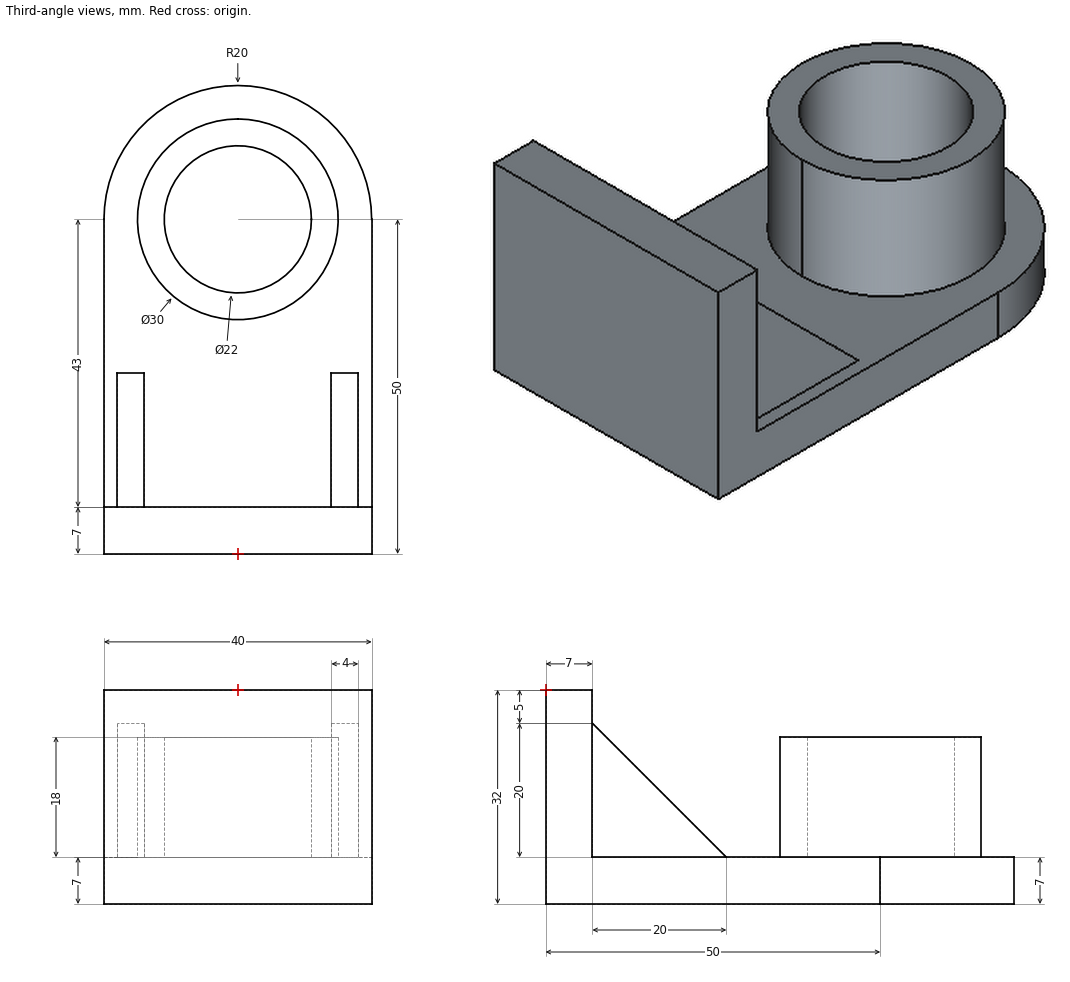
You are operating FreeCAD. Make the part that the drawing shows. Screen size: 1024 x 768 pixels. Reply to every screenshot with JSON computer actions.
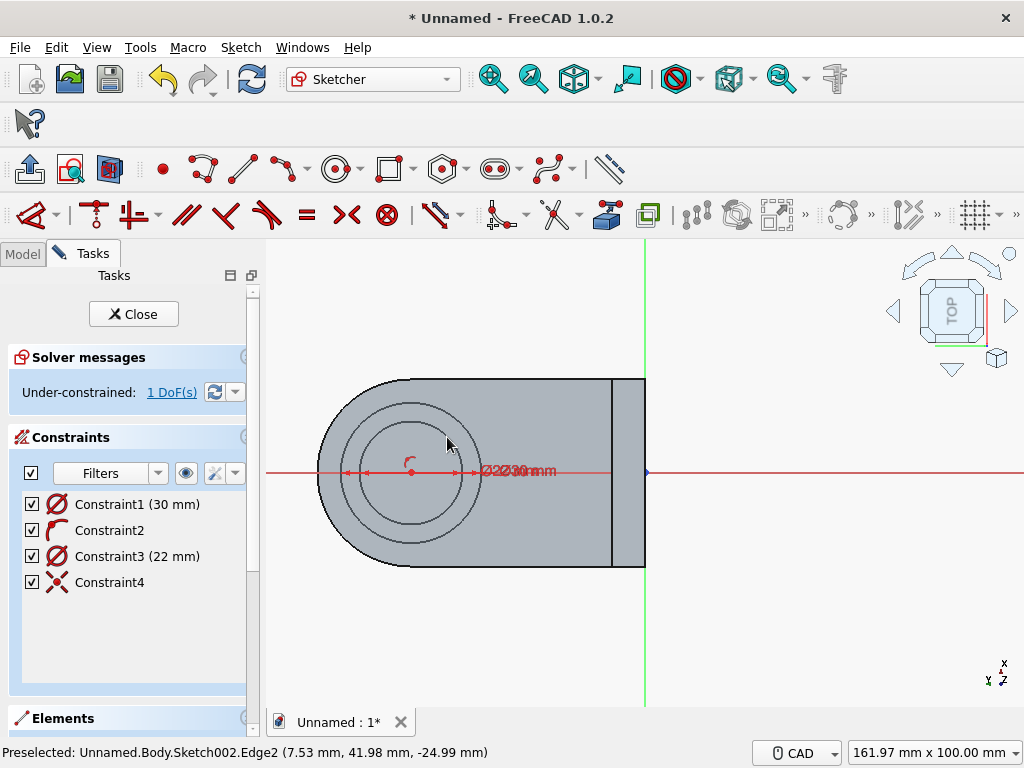
{"action": "left_click", "coordinate": [32, 216]}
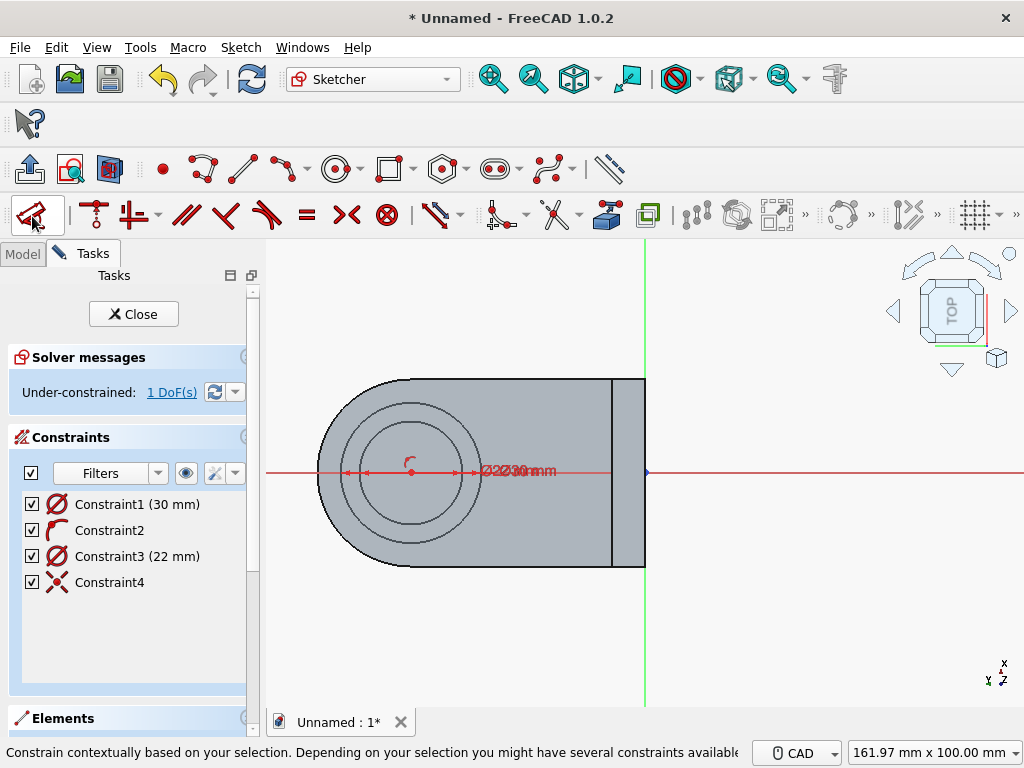
{"action": "left_click", "coordinate": [411, 473]}
{"action": "left_click", "coordinate": [528, 439]}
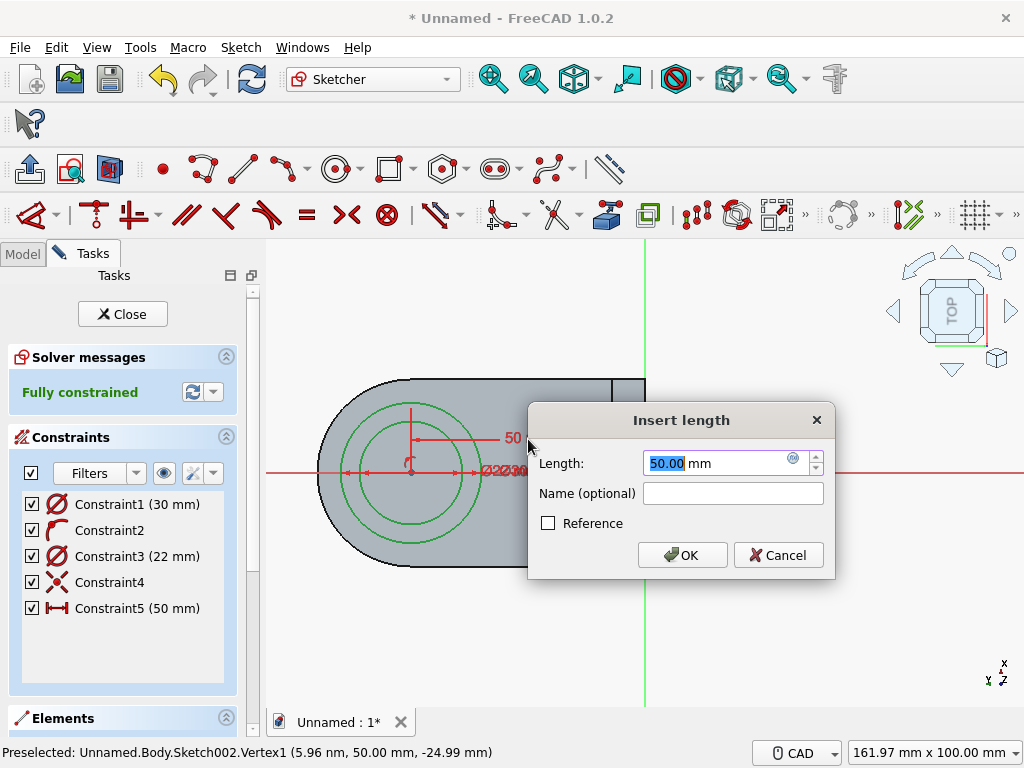
{"action": "type", "text": "50"}
{"action": "key", "text": "Return"}
{"action": "key", "text": "Escape"}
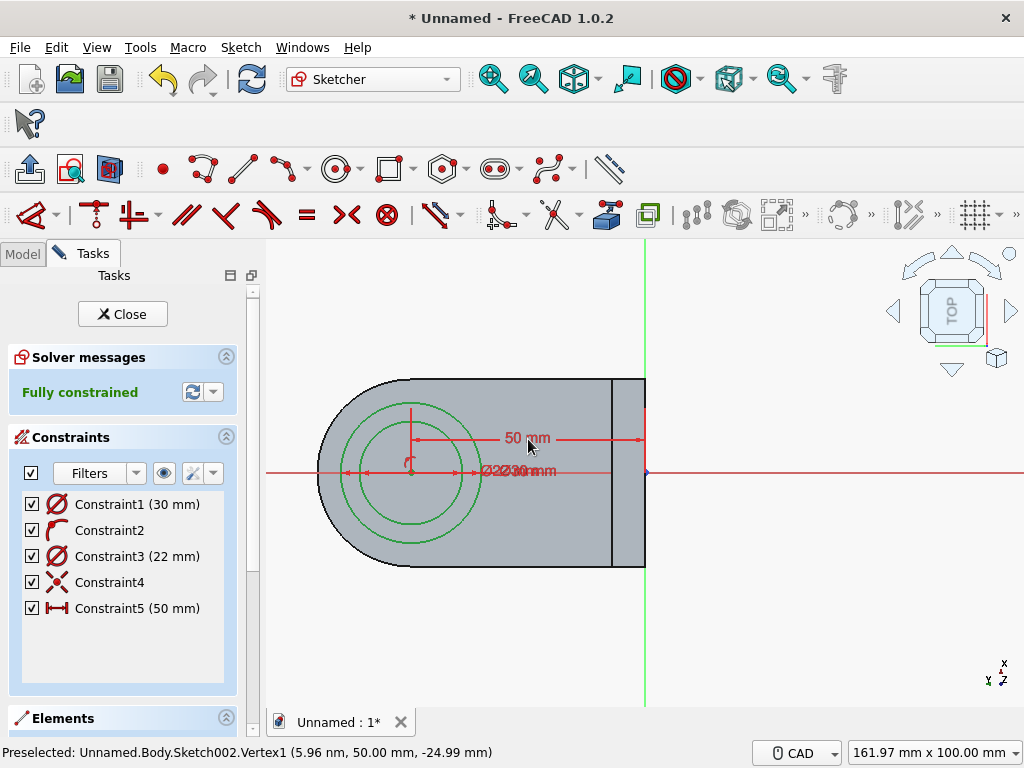
{"action": "left_click", "coordinate": [123, 314]}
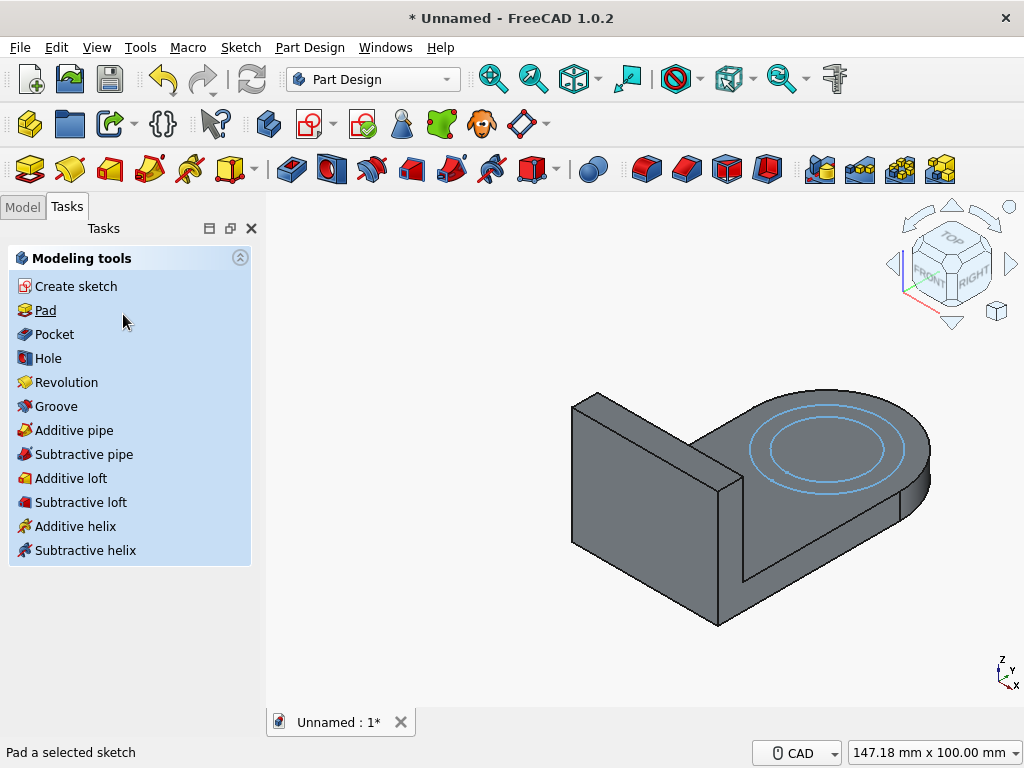
{"action": "left_click", "coordinate": [30, 170]}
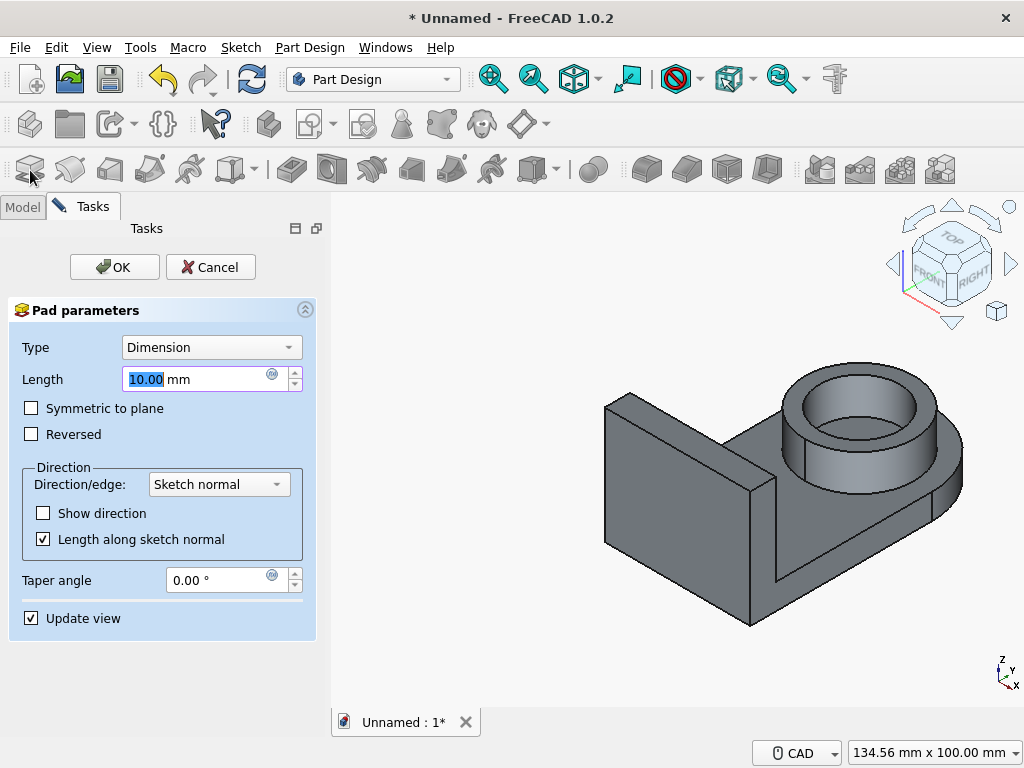
{"action": "type", "text": "18"}
{"action": "key", "text": "Tab"}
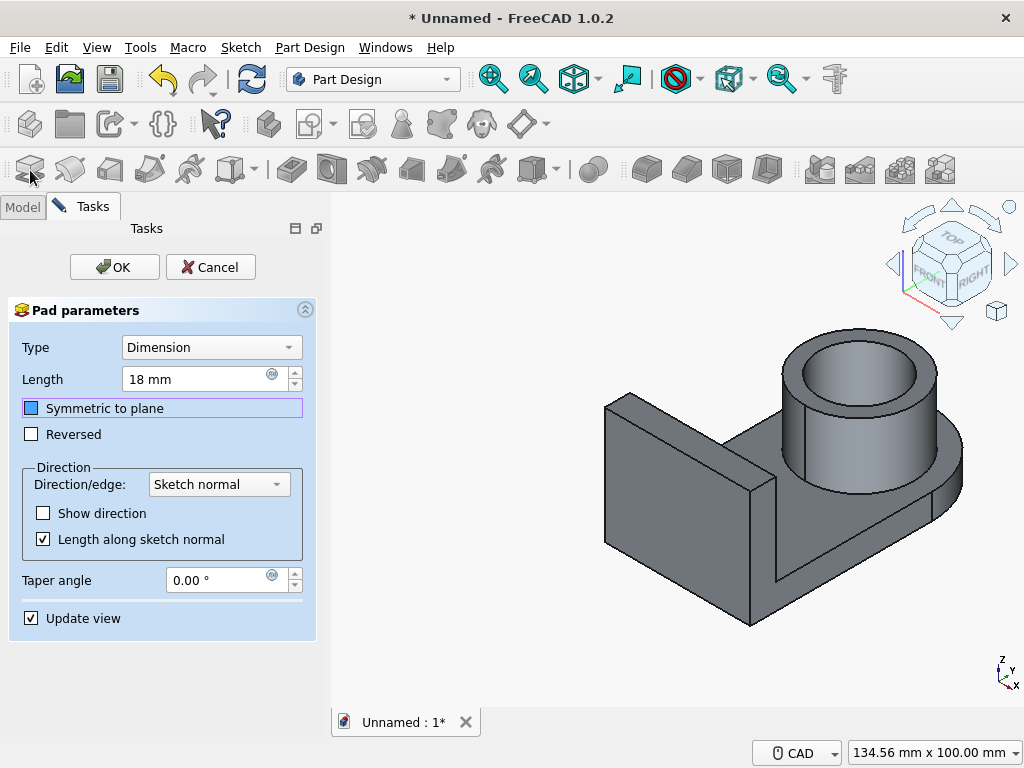
{"action": "left_click", "coordinate": [115, 267]}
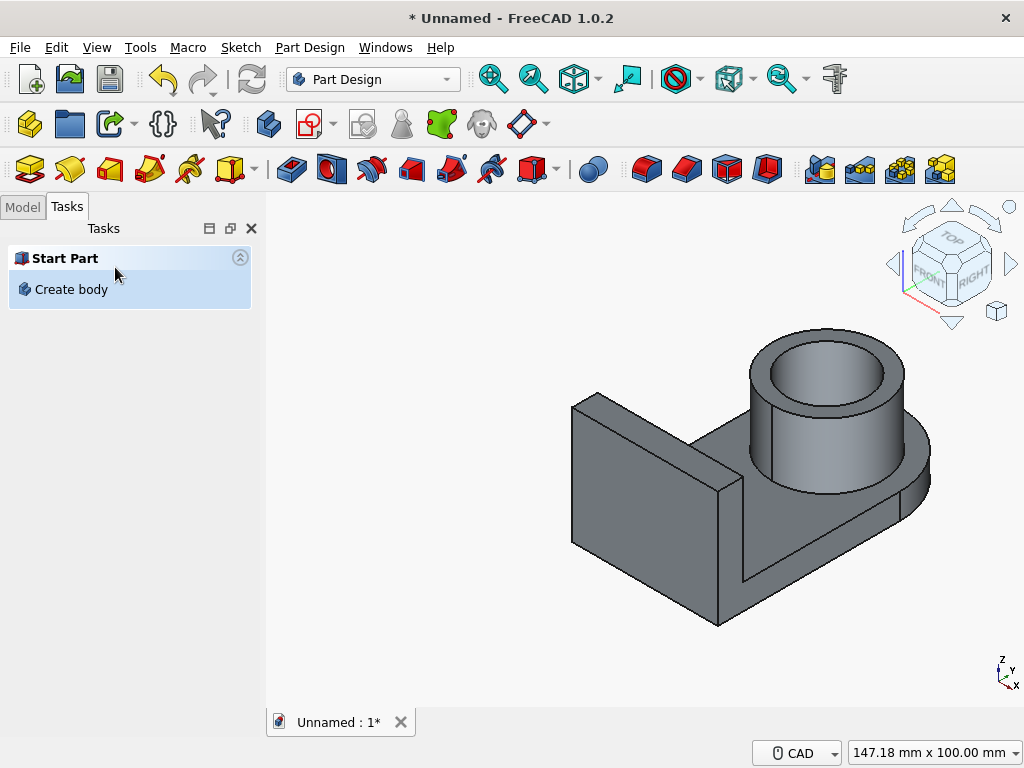
{"action": "left_click", "coordinate": [23, 206]}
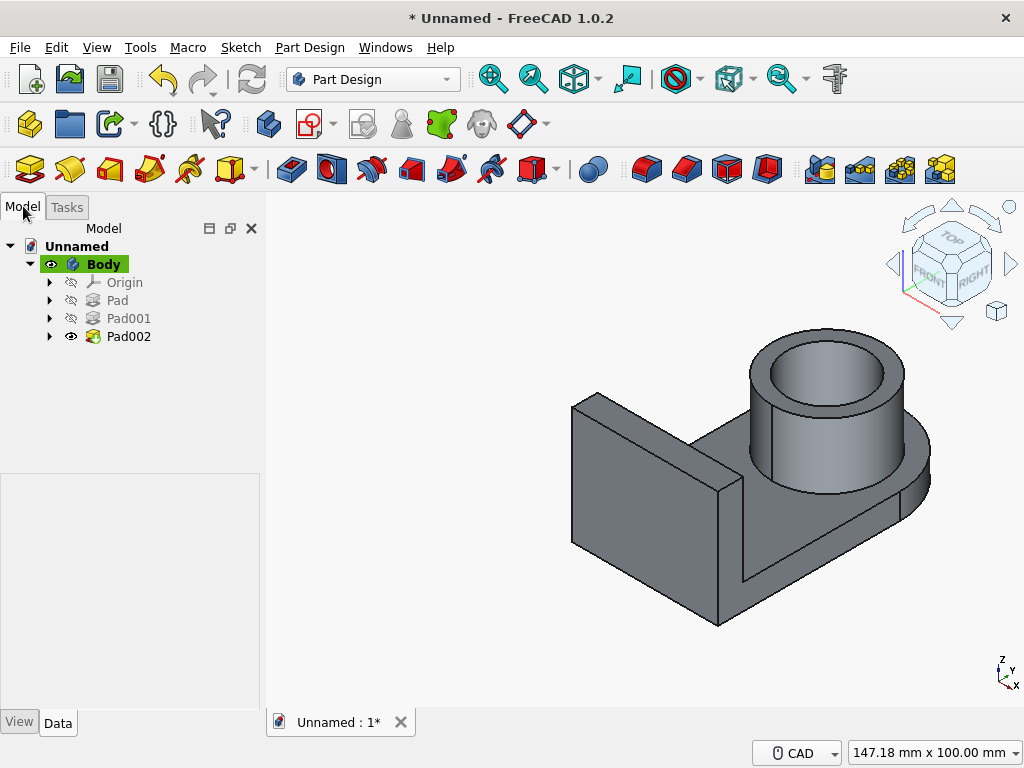
{"action": "left_click", "coordinate": [50, 282]}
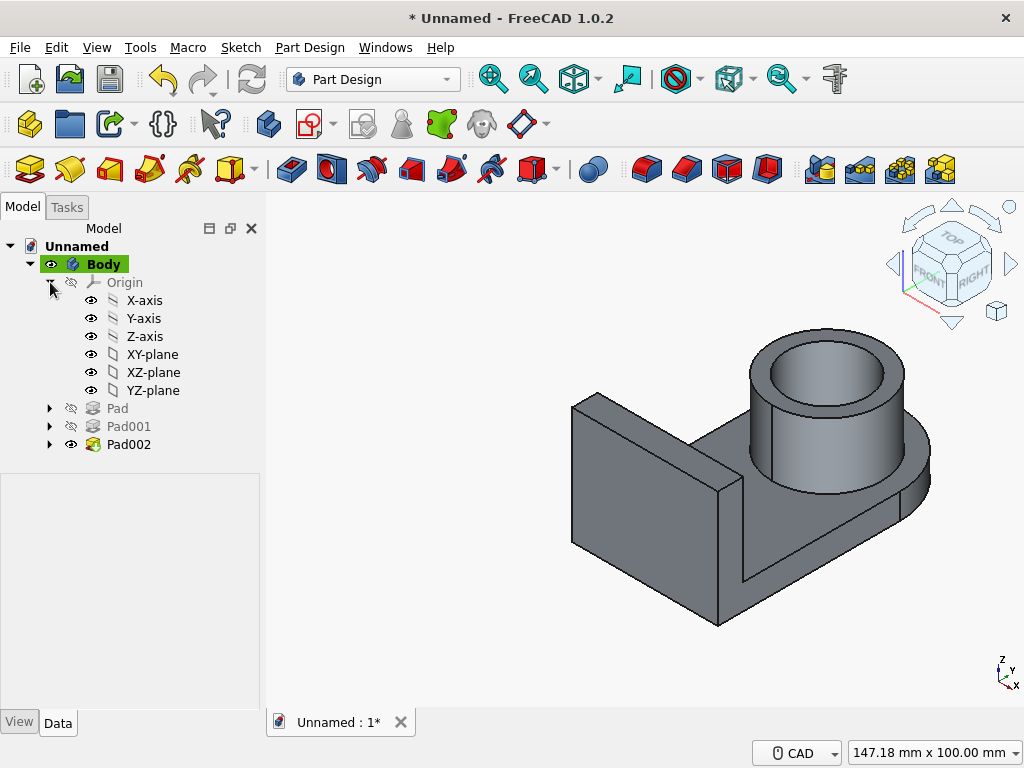
{"action": "left_click", "coordinate": [136, 390]}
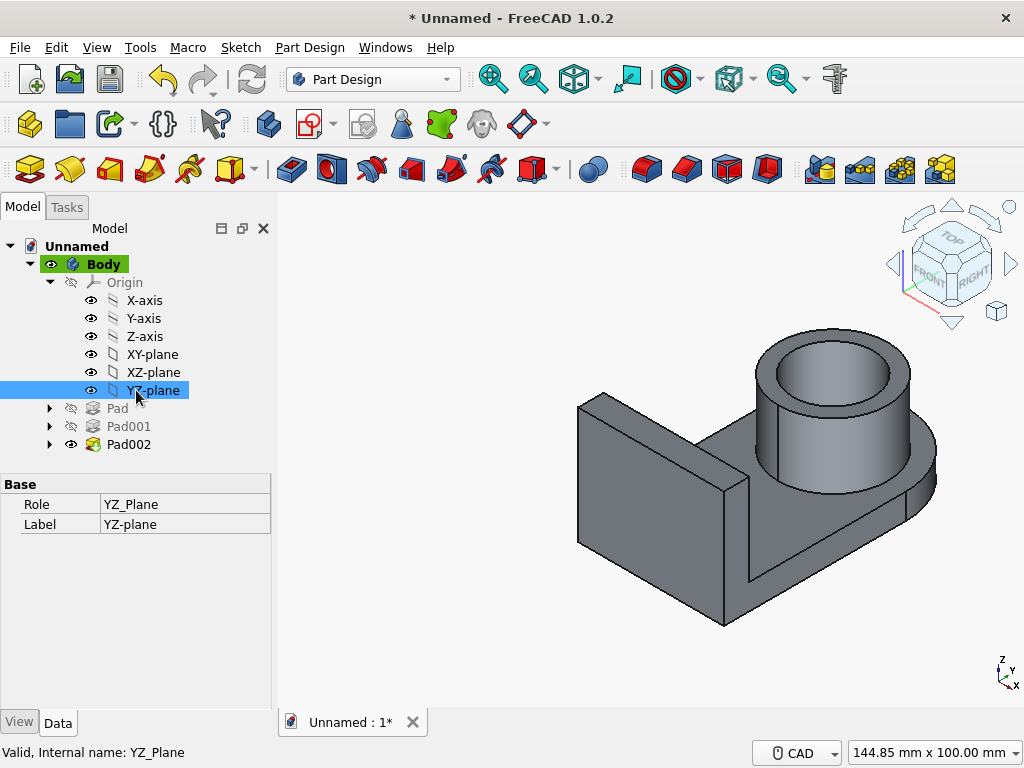
{"action": "left_click", "coordinate": [522, 124]}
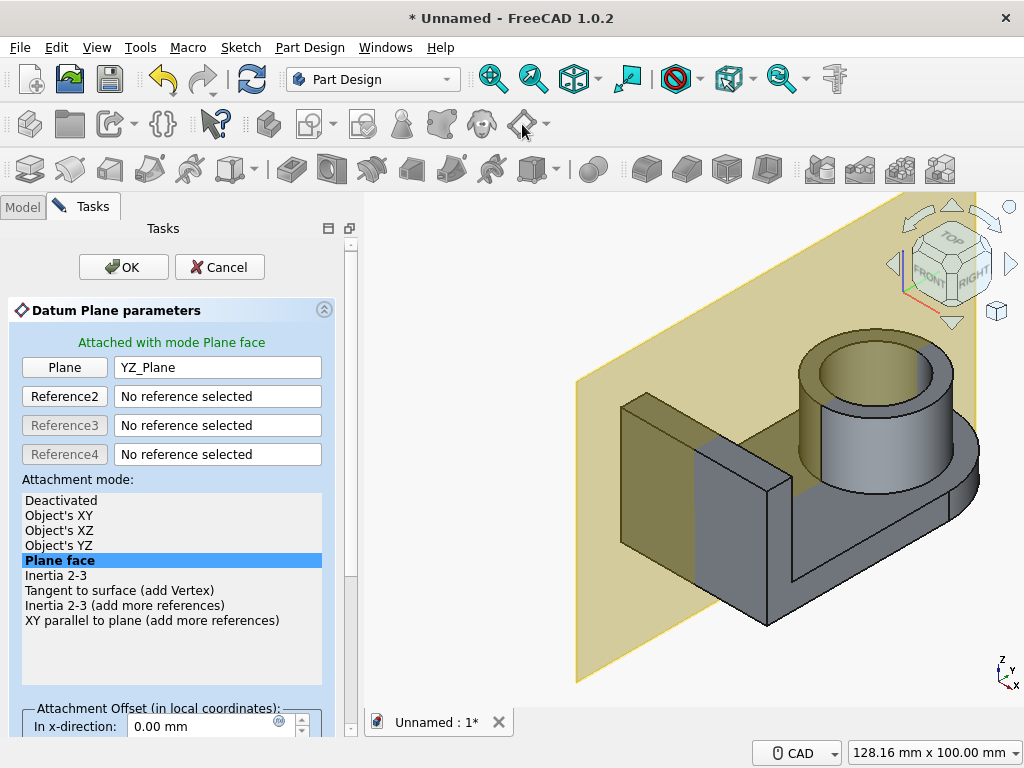
{"action": "scroll", "coordinate": [351, 487], "scroll_direction": "down", "scroll_amount": 3}